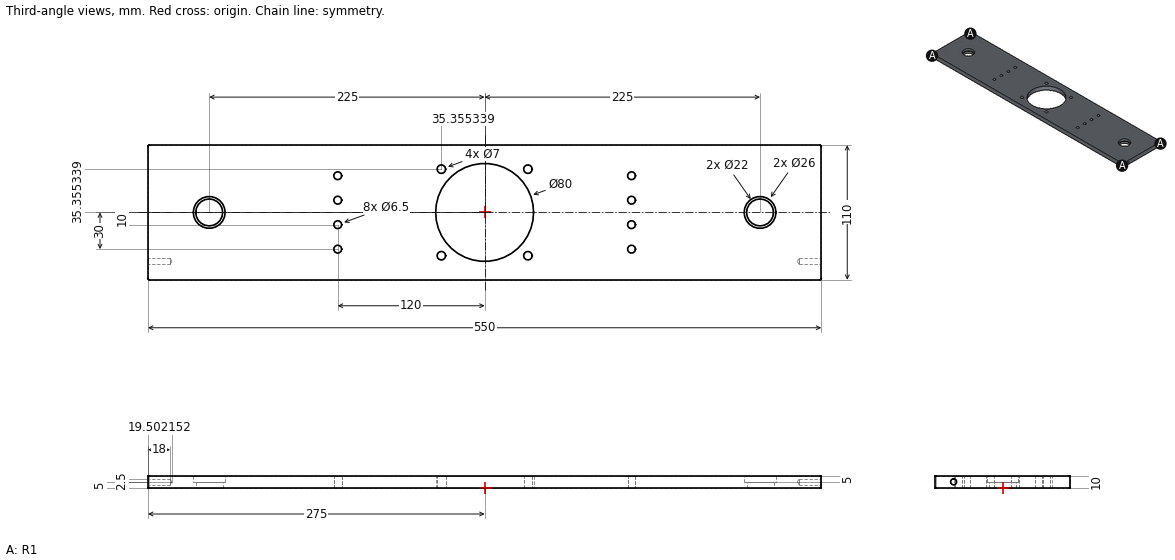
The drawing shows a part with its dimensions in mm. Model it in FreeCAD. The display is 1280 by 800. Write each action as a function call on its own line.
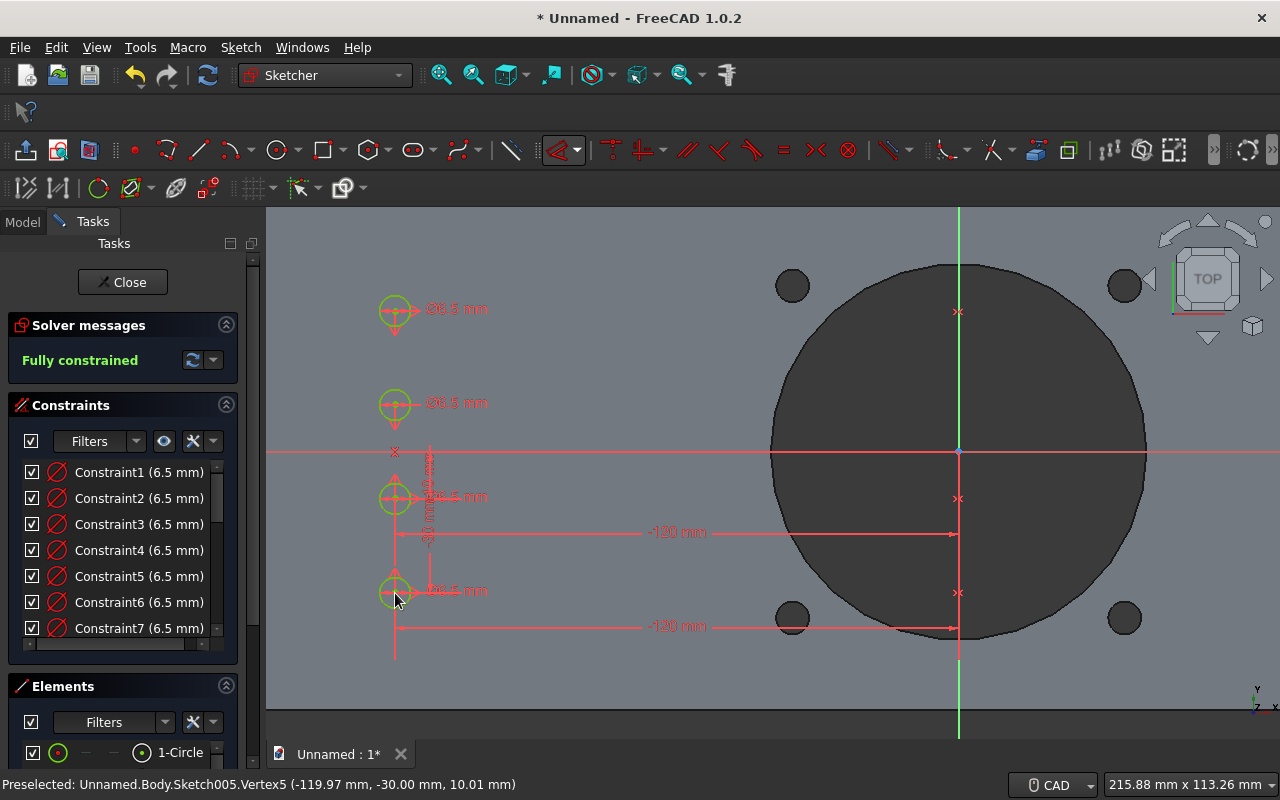
click(123, 282)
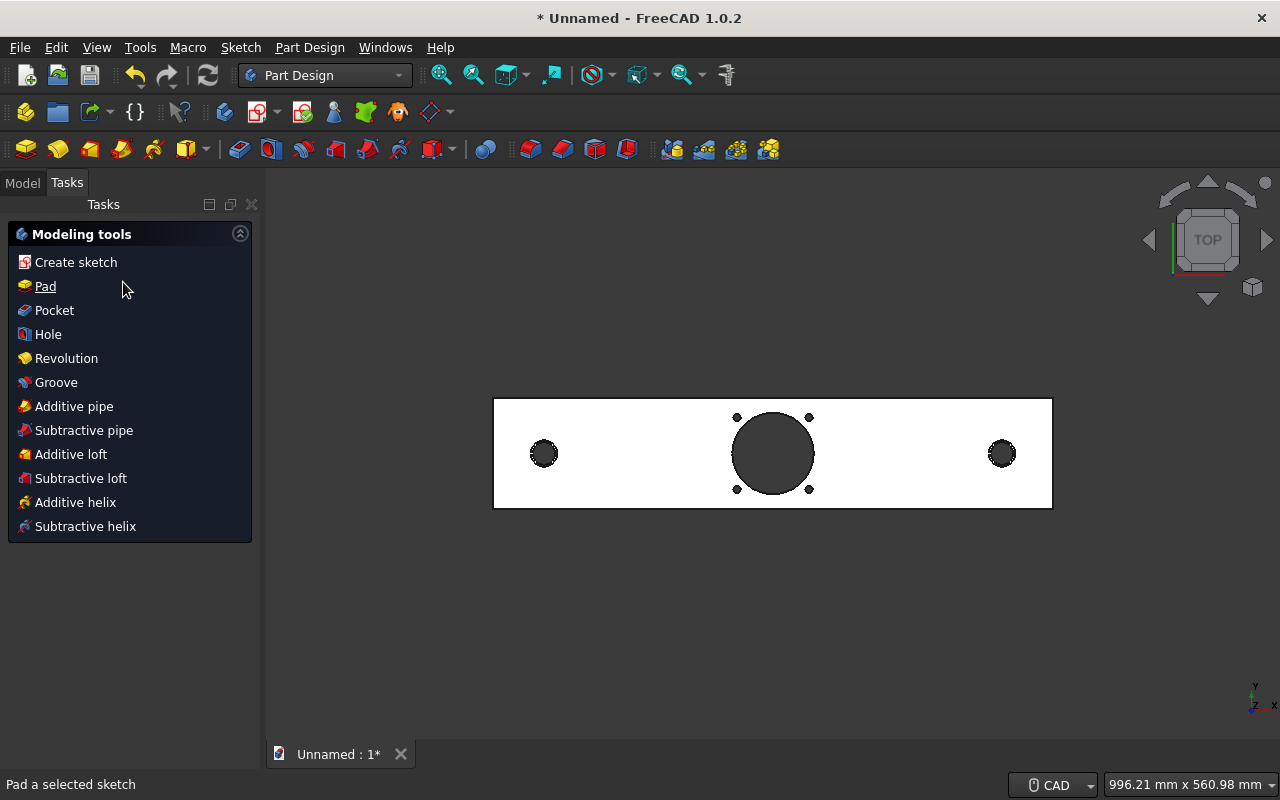
click(240, 150)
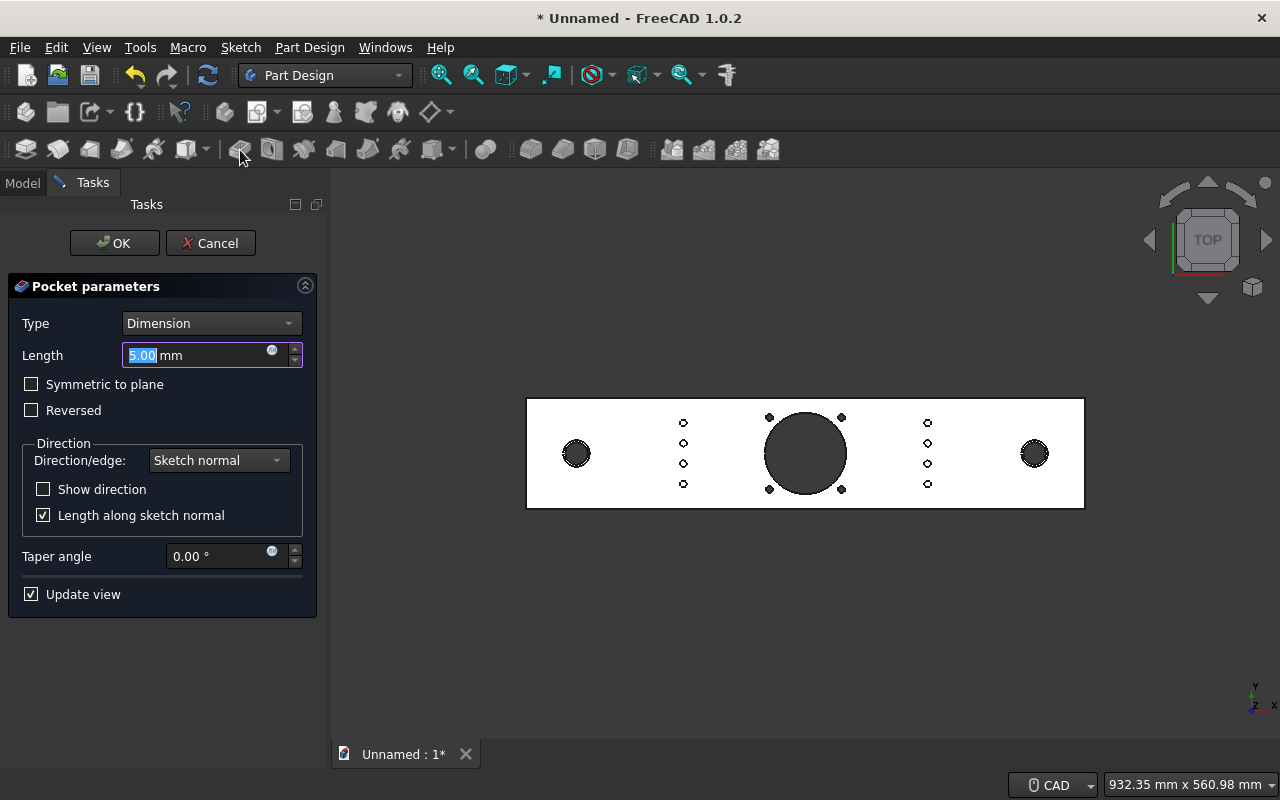
click(212, 324)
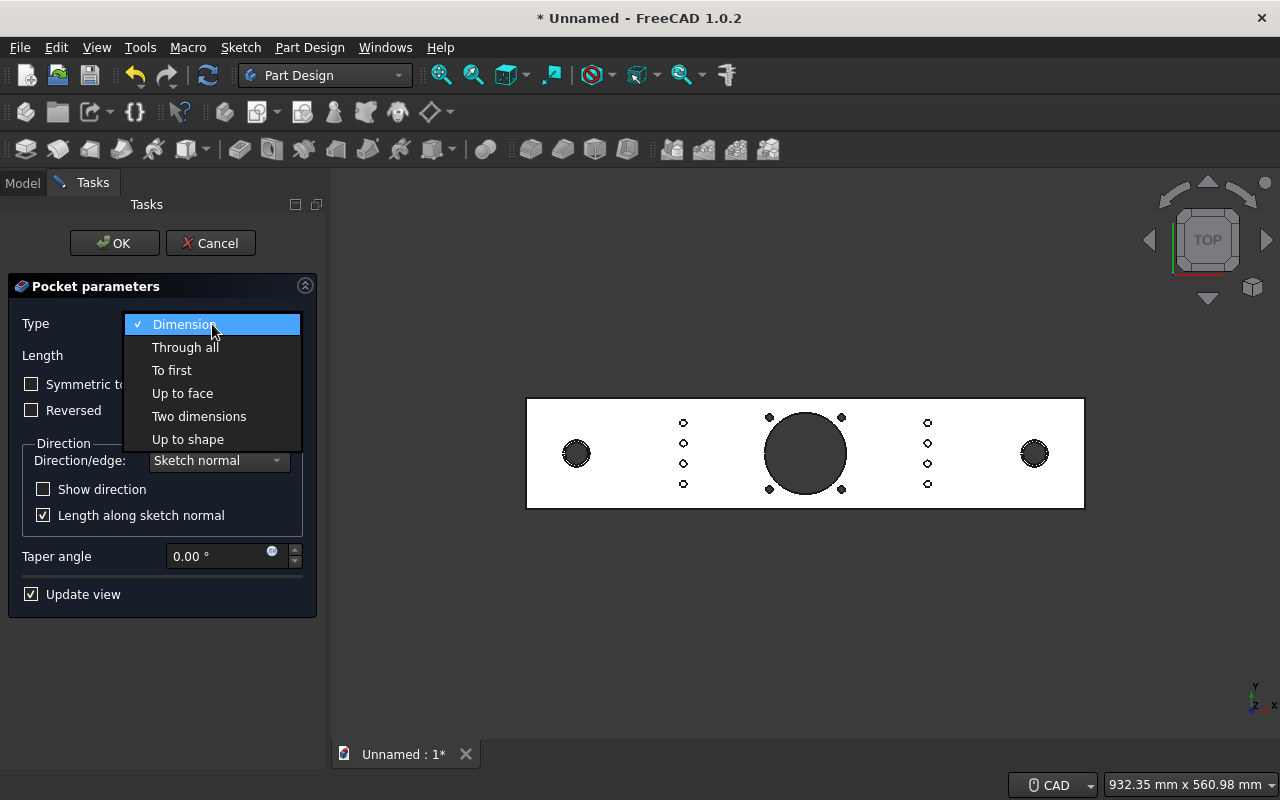
click(212, 348)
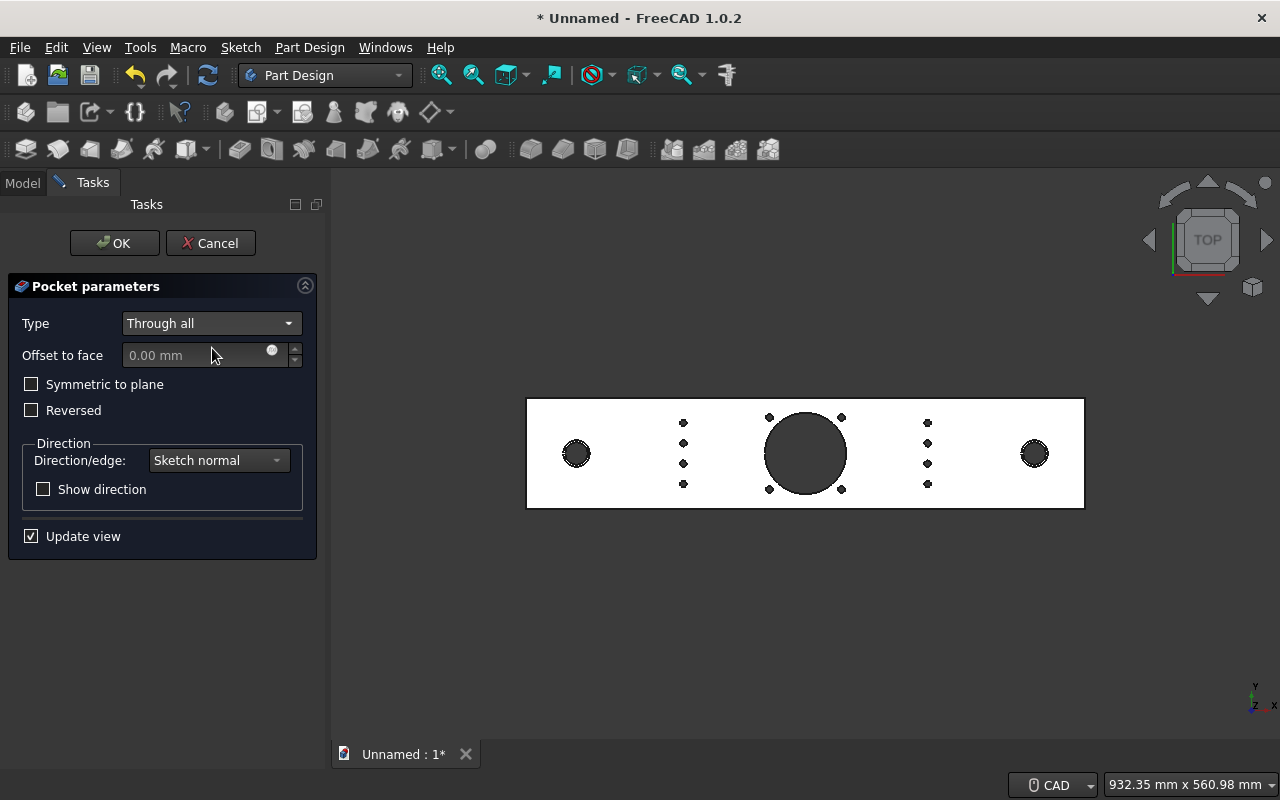
click(115, 243)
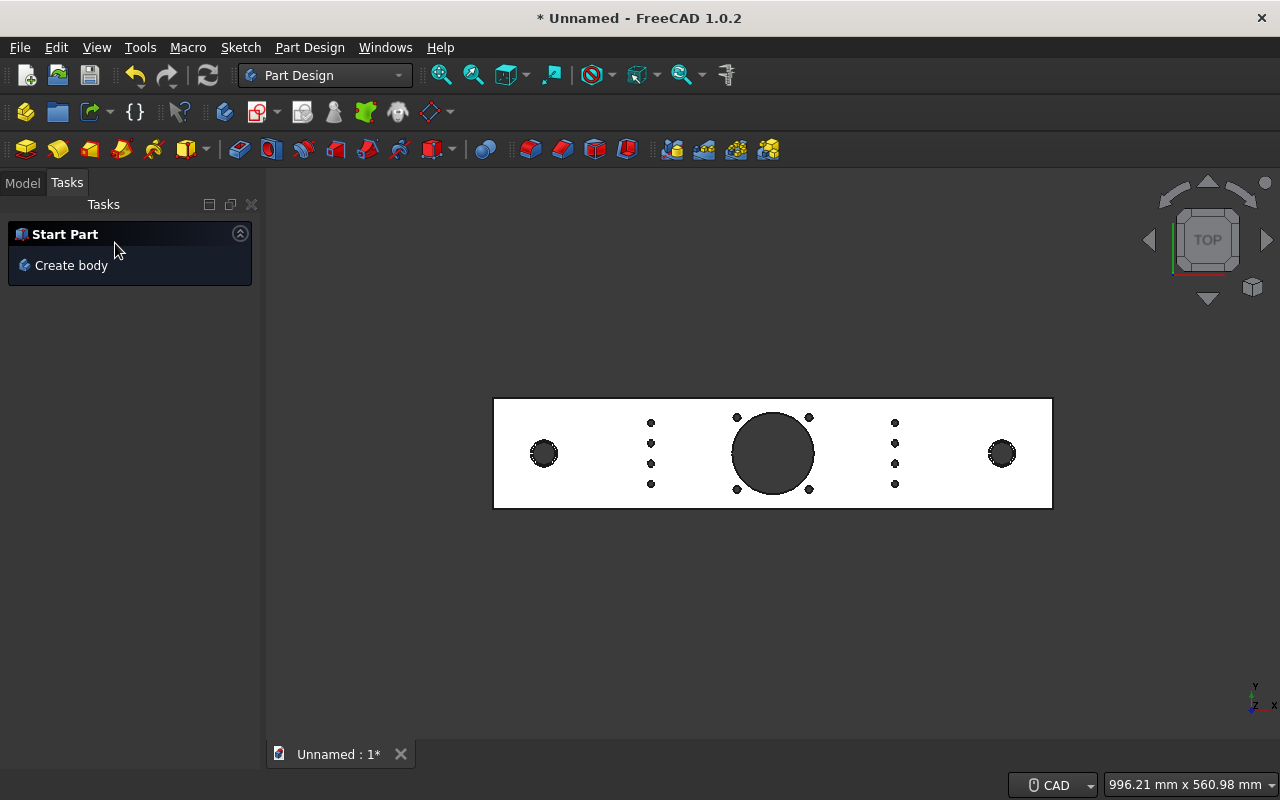
scroll(493, 397, up, 7)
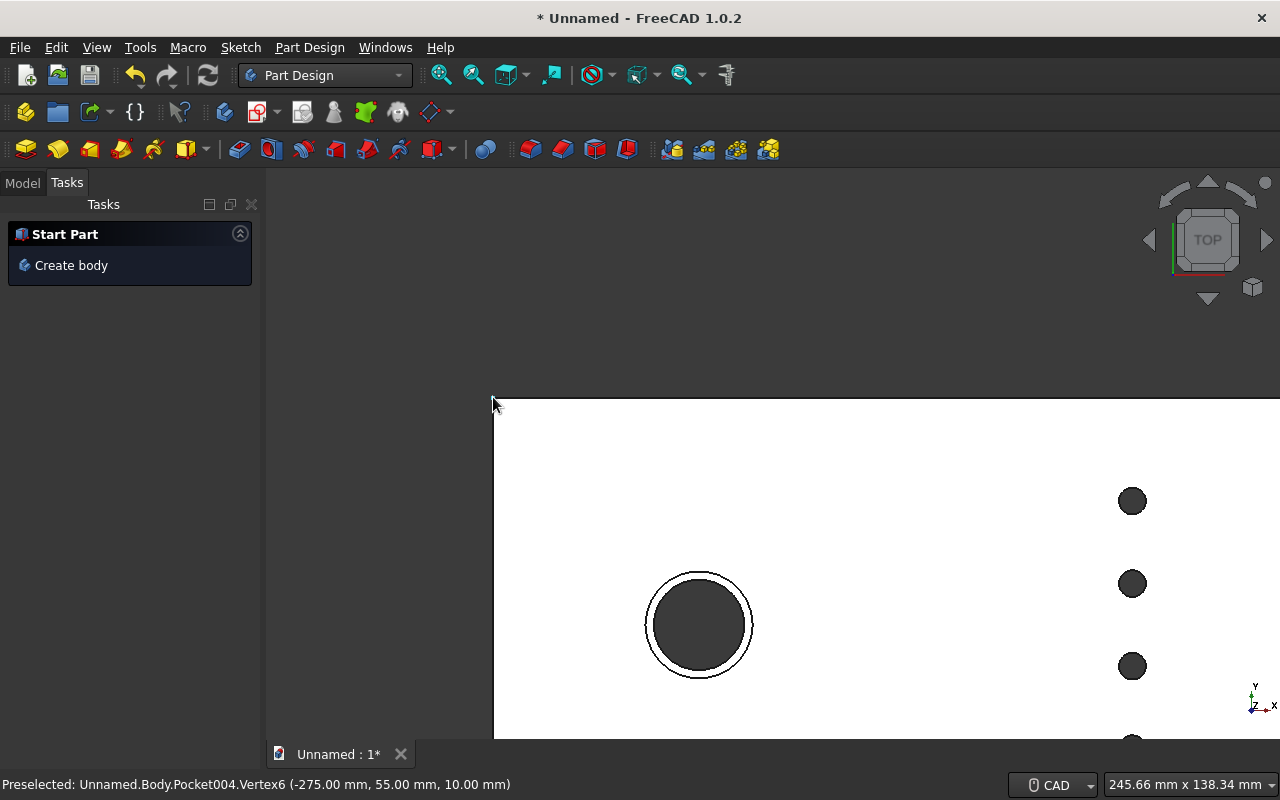
key(v)
key(f)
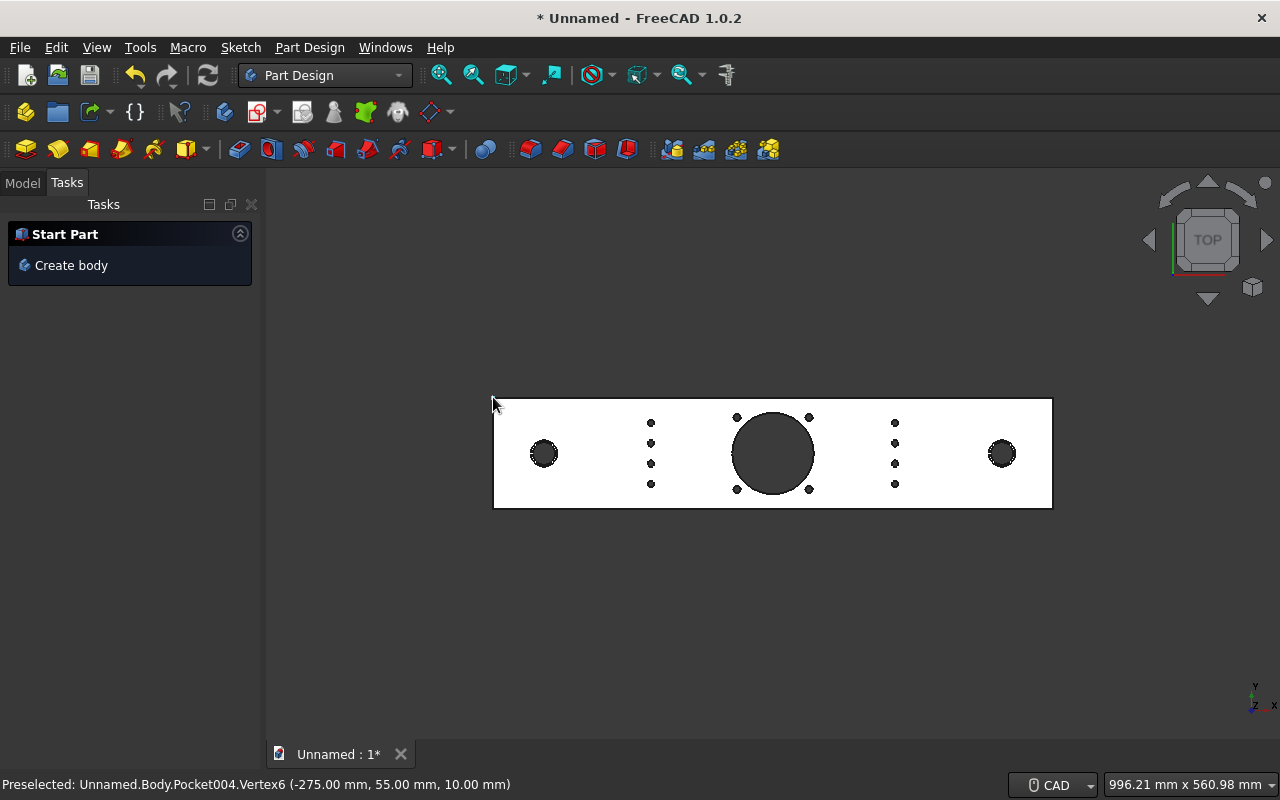
key(0)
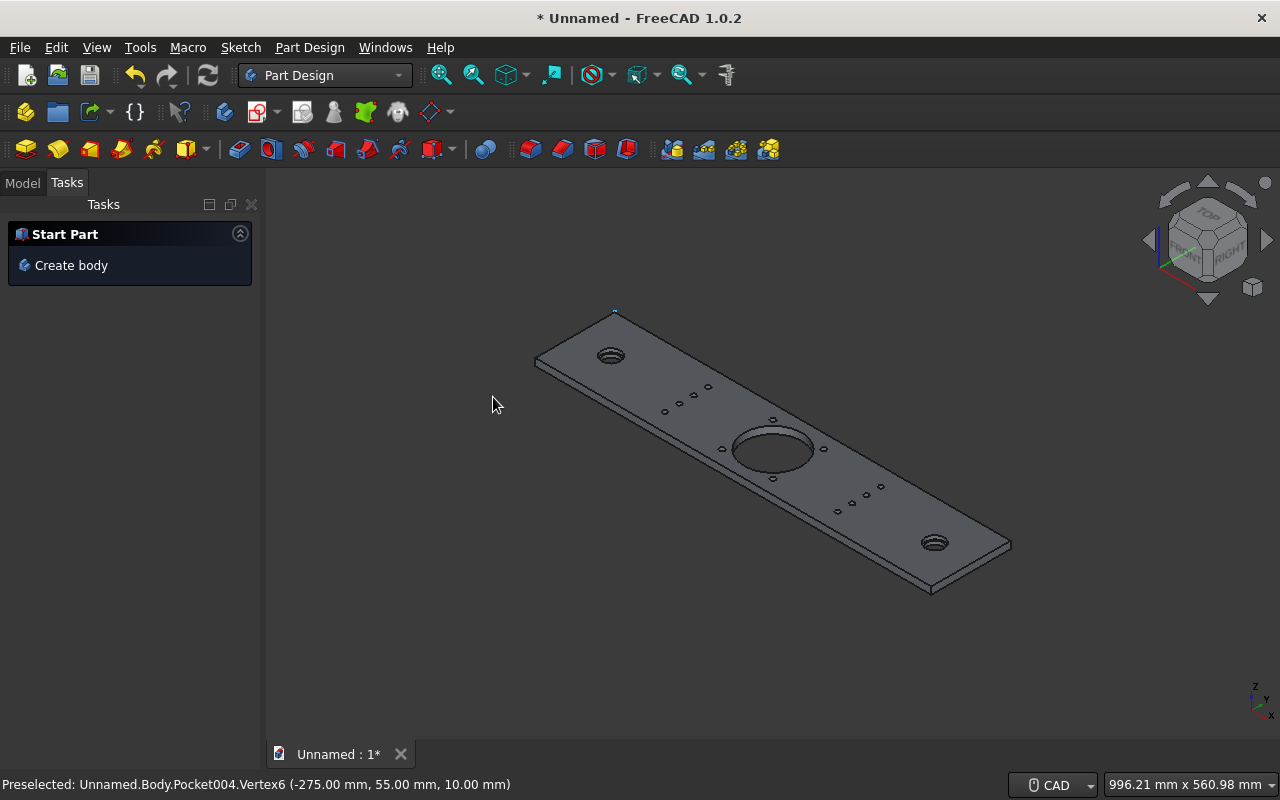
click(931, 592)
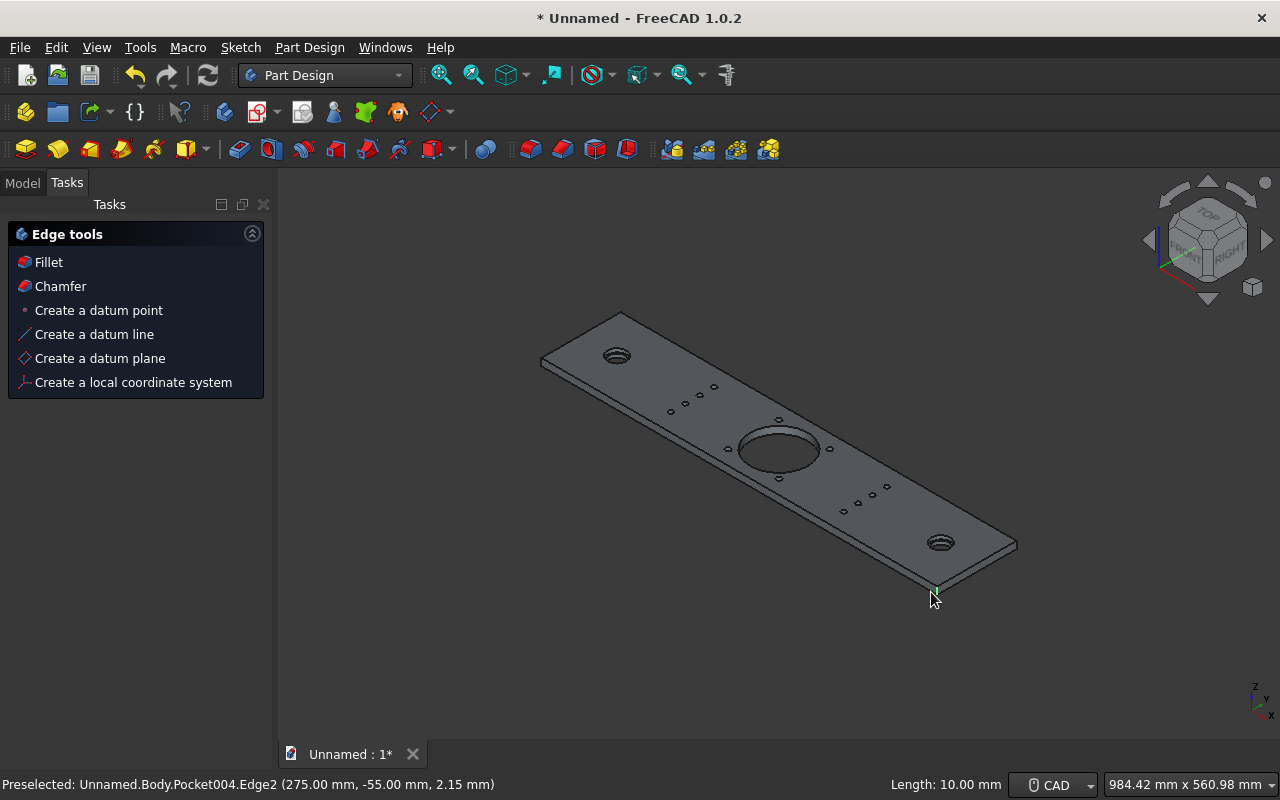
scroll(621, 315, up, 7)